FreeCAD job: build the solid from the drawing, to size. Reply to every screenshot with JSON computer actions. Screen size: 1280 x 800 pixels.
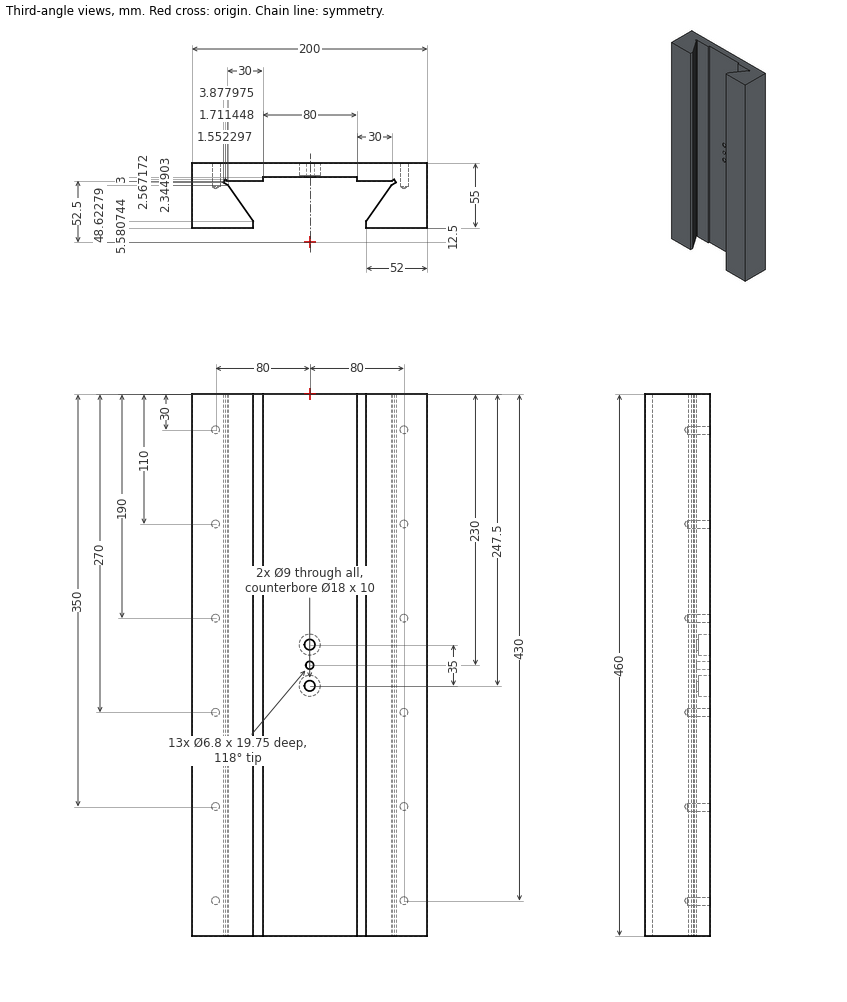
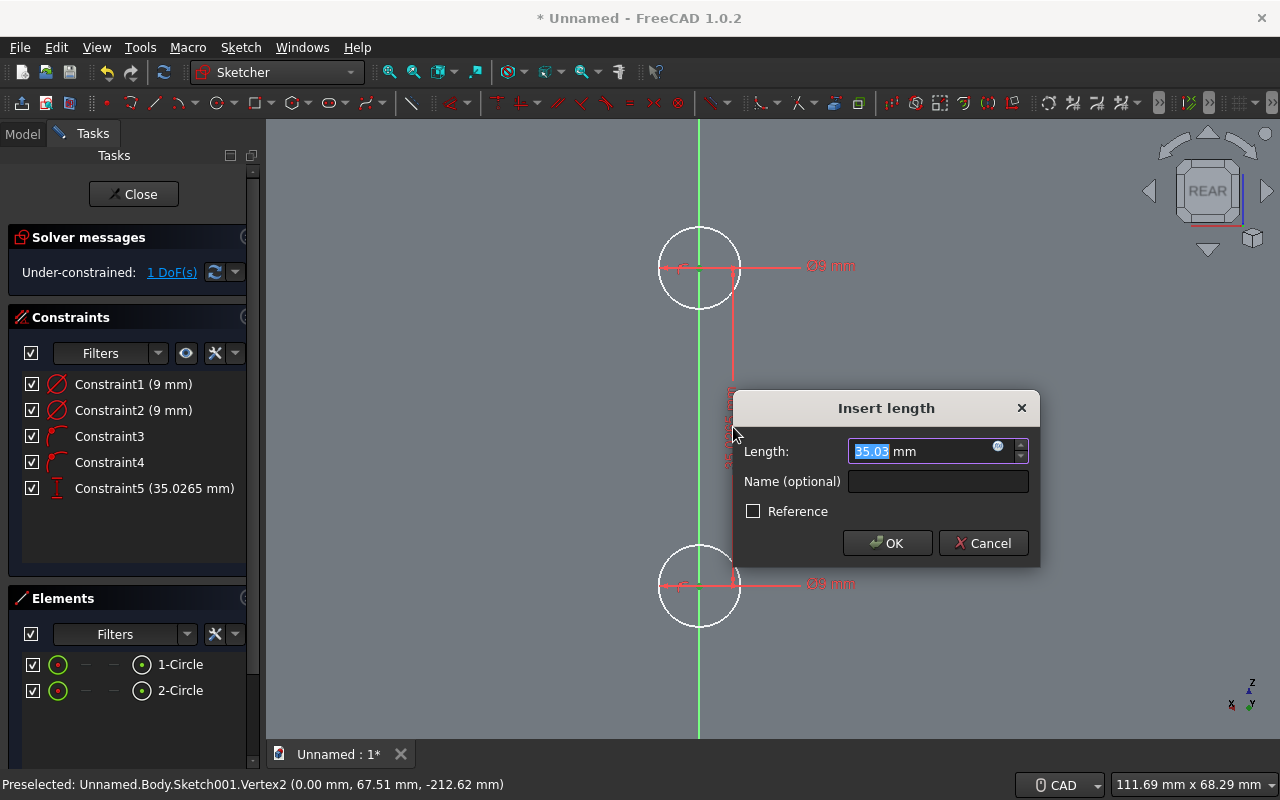
{"action": "type", "text": "35"}
{"action": "key", "text": "Return"}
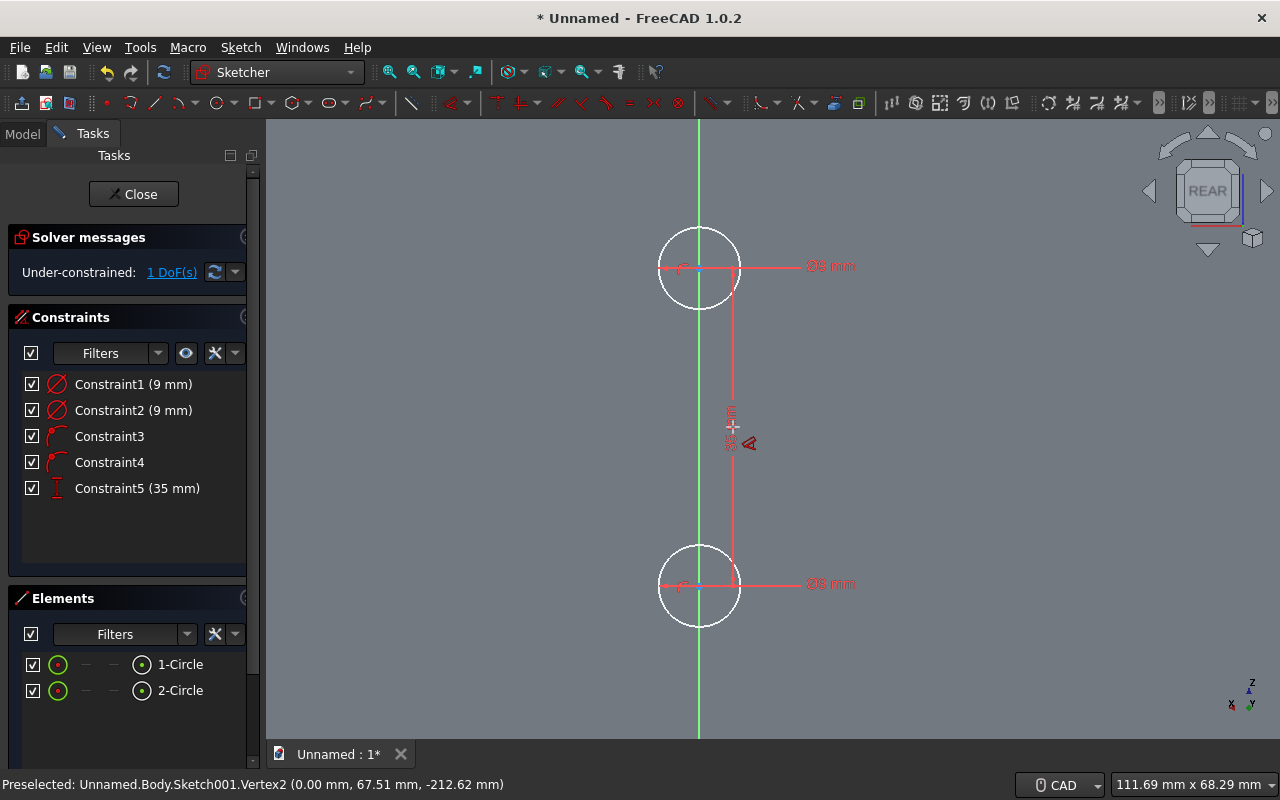
{"action": "left_click", "coordinate": [699, 586]}
{"action": "left_click", "coordinate": [733, 366]}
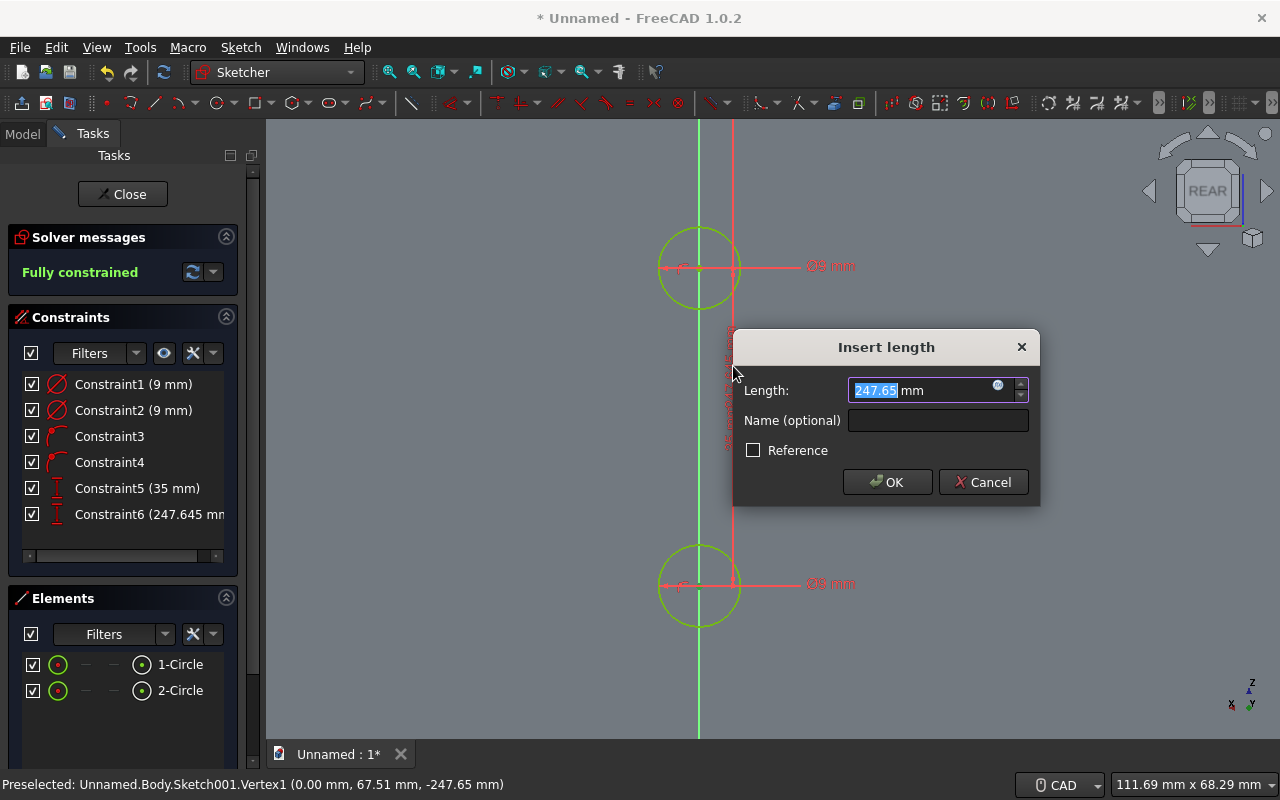
{"action": "type", "text": "247.5"}
{"action": "key", "text": "Return"}
{"action": "key", "text": "Escape"}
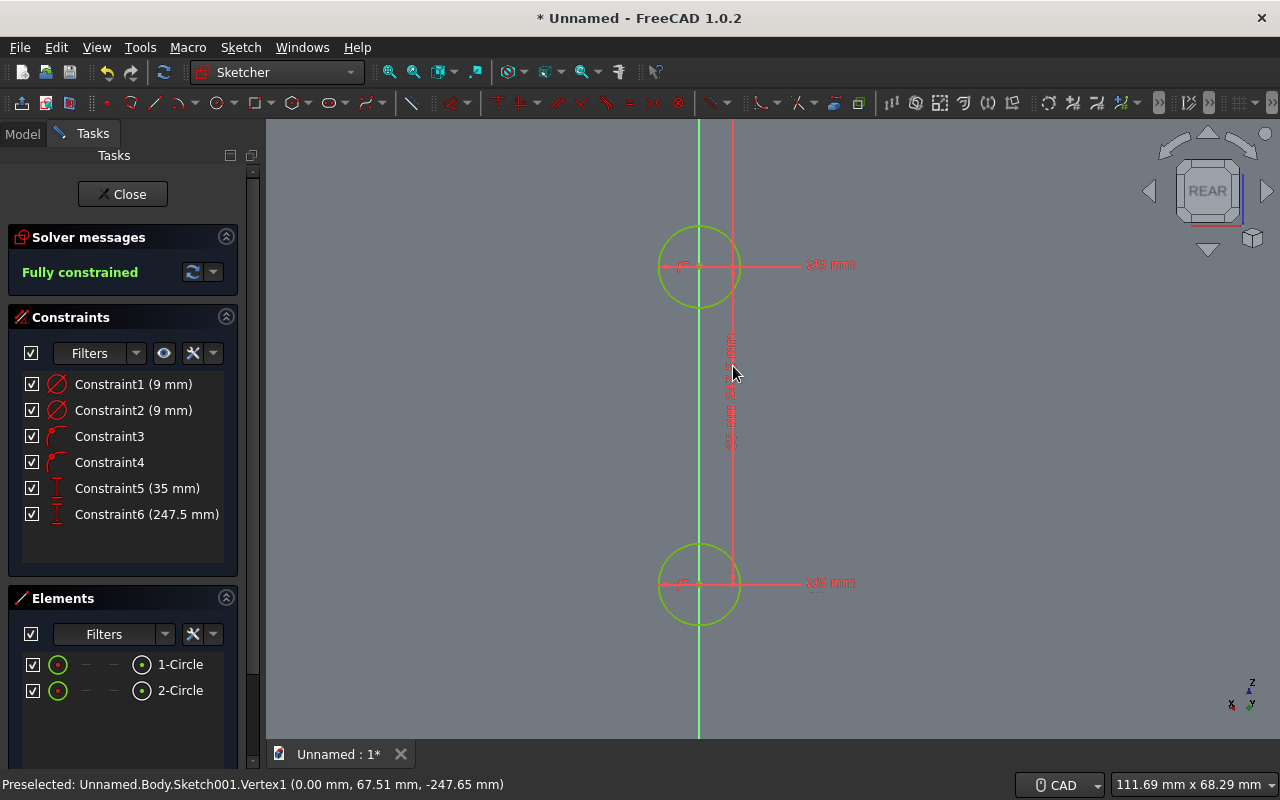
{"action": "left_click", "coordinate": [123, 194]}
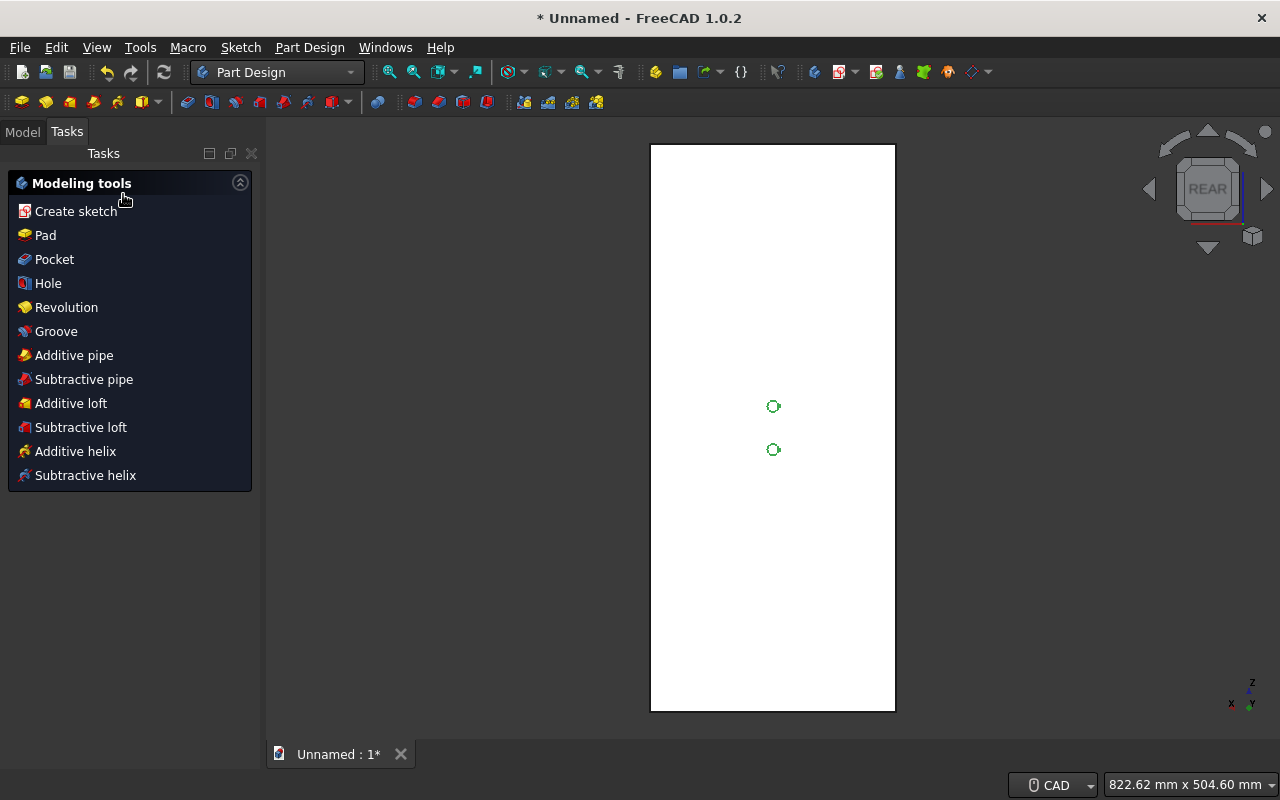
{"action": "left_click", "coordinate": [212, 102]}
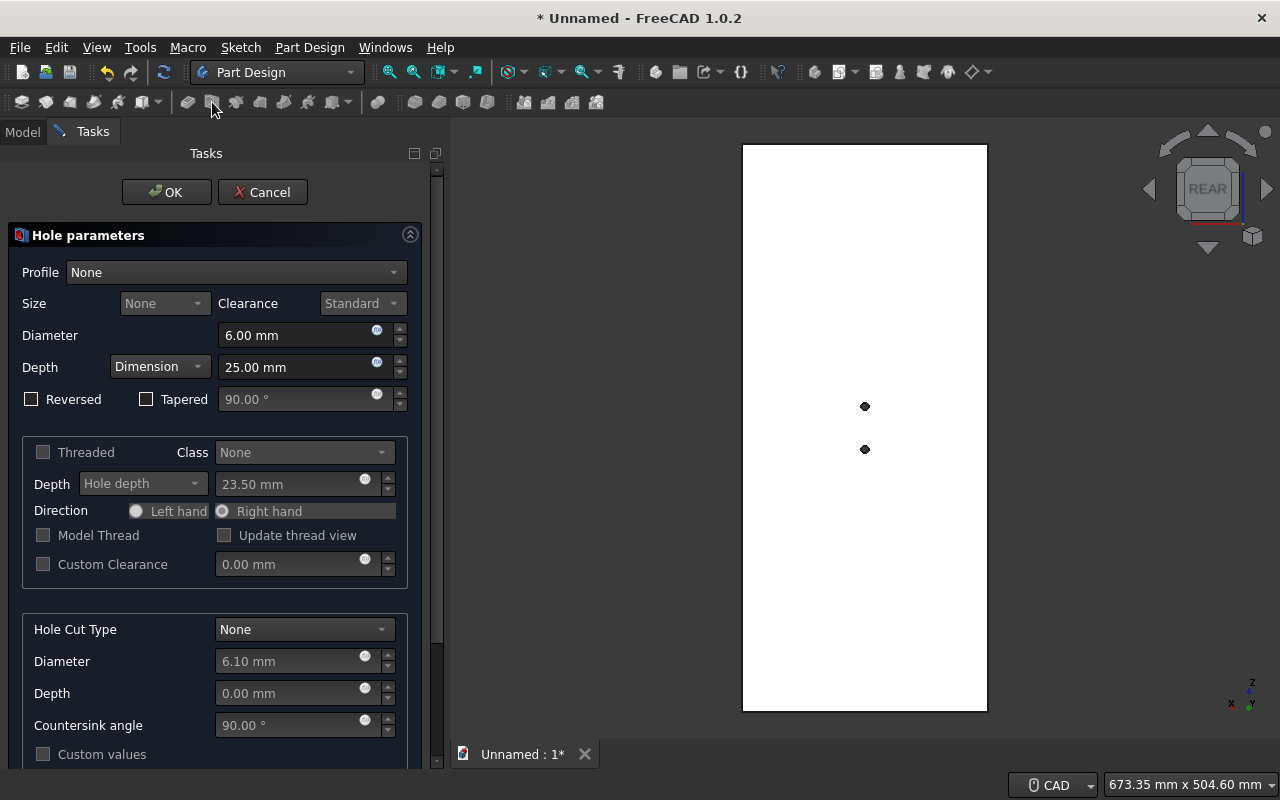
{"action": "triple_click", "coordinate": [305, 335]}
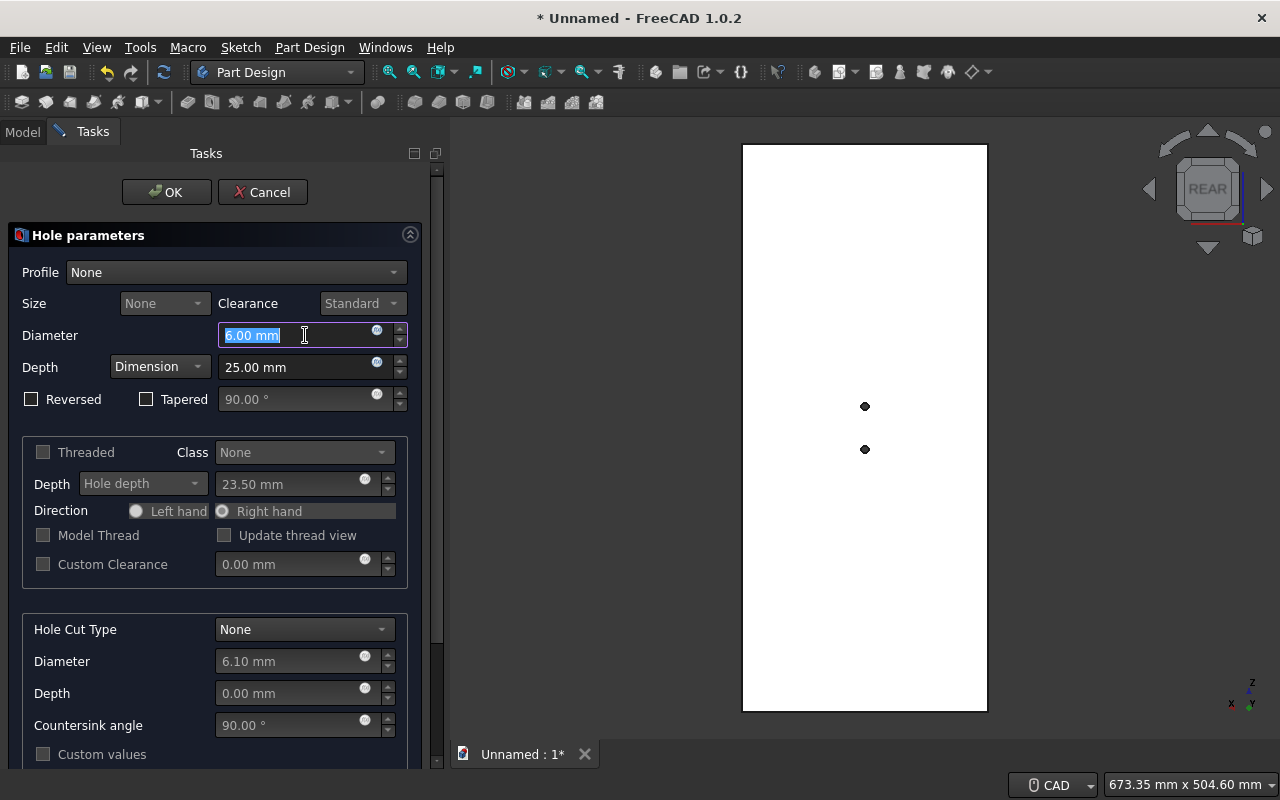
{"action": "type", "text": "9"}
{"action": "key", "text": "Tab"}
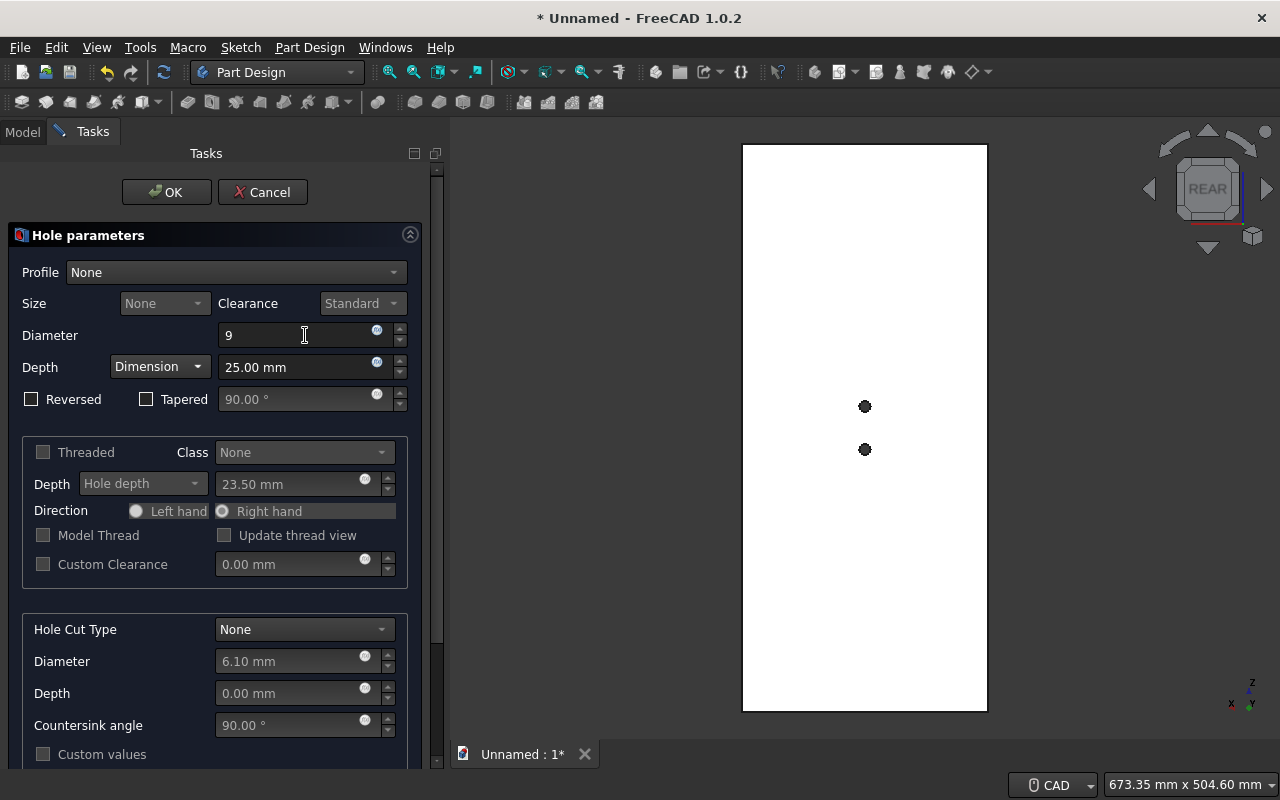
{"action": "left_click", "coordinate": [161, 366]}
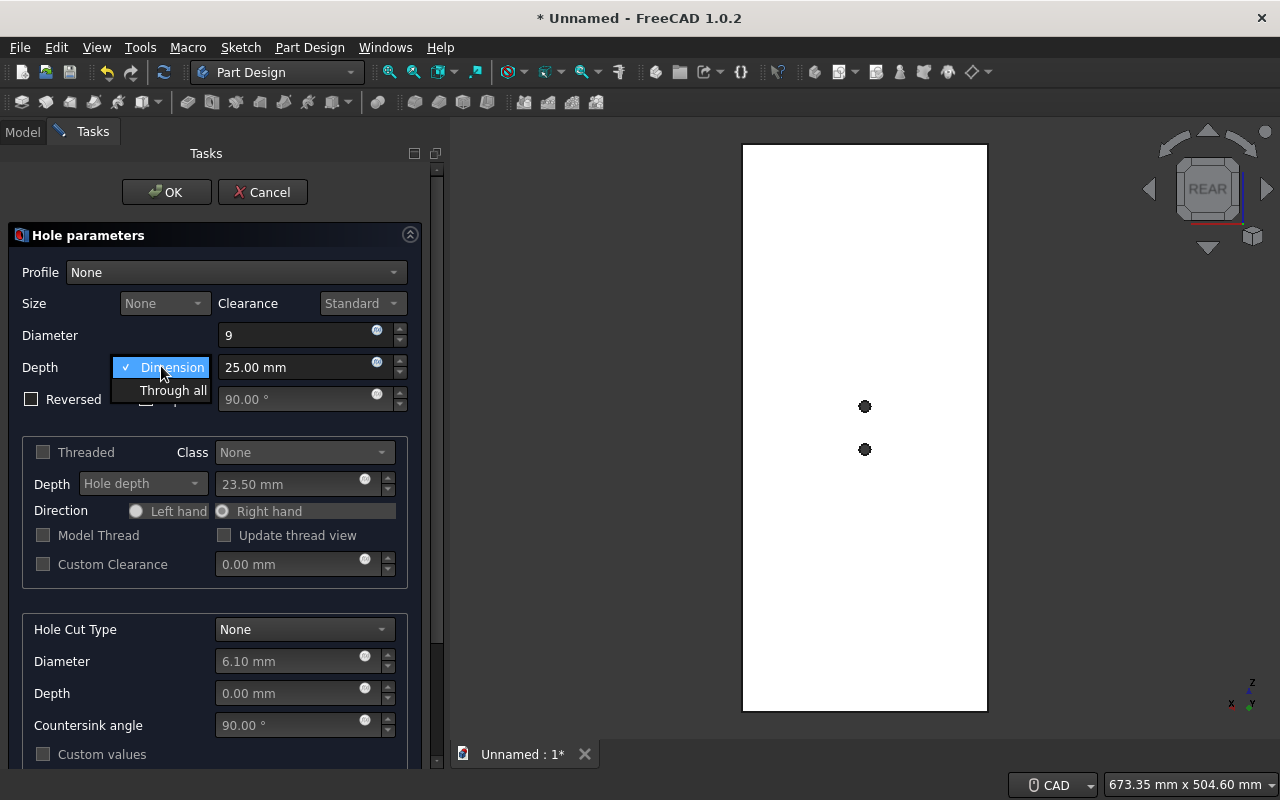
{"action": "left_click", "coordinate": [160, 390]}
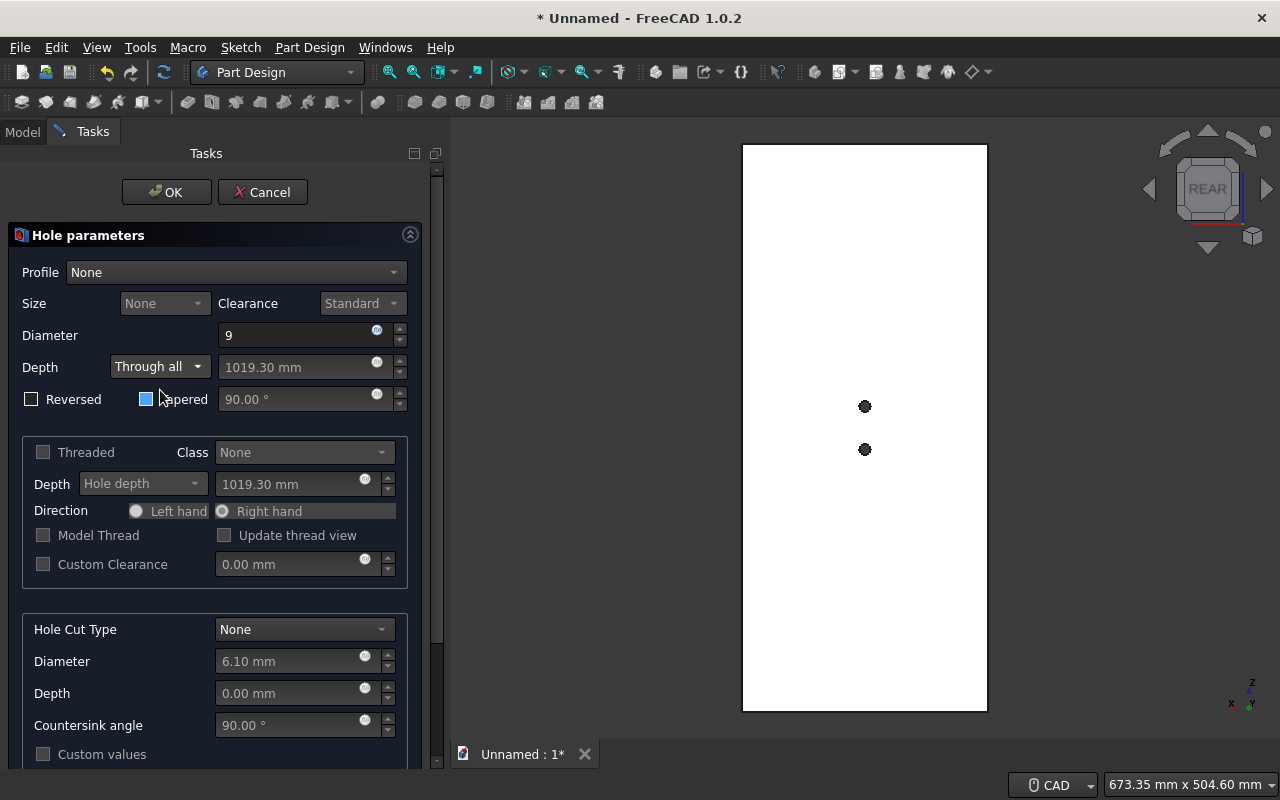
{"action": "left_click", "coordinate": [306, 630]}